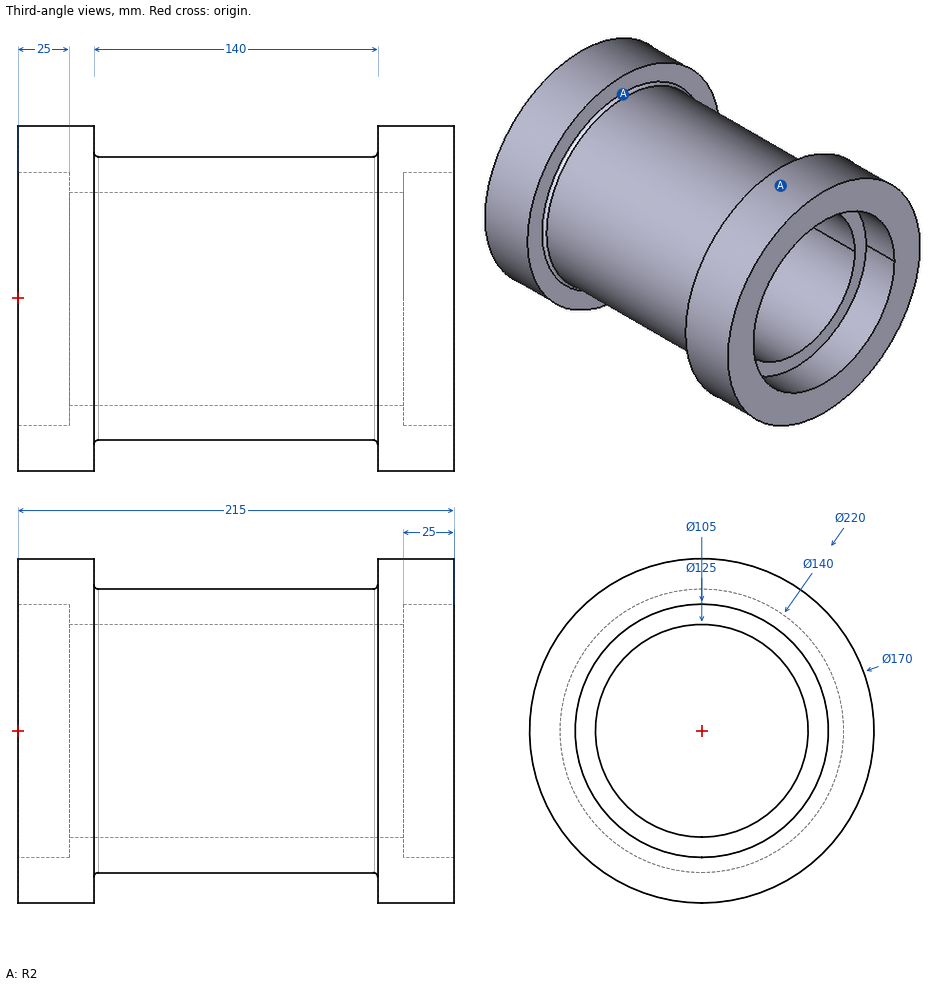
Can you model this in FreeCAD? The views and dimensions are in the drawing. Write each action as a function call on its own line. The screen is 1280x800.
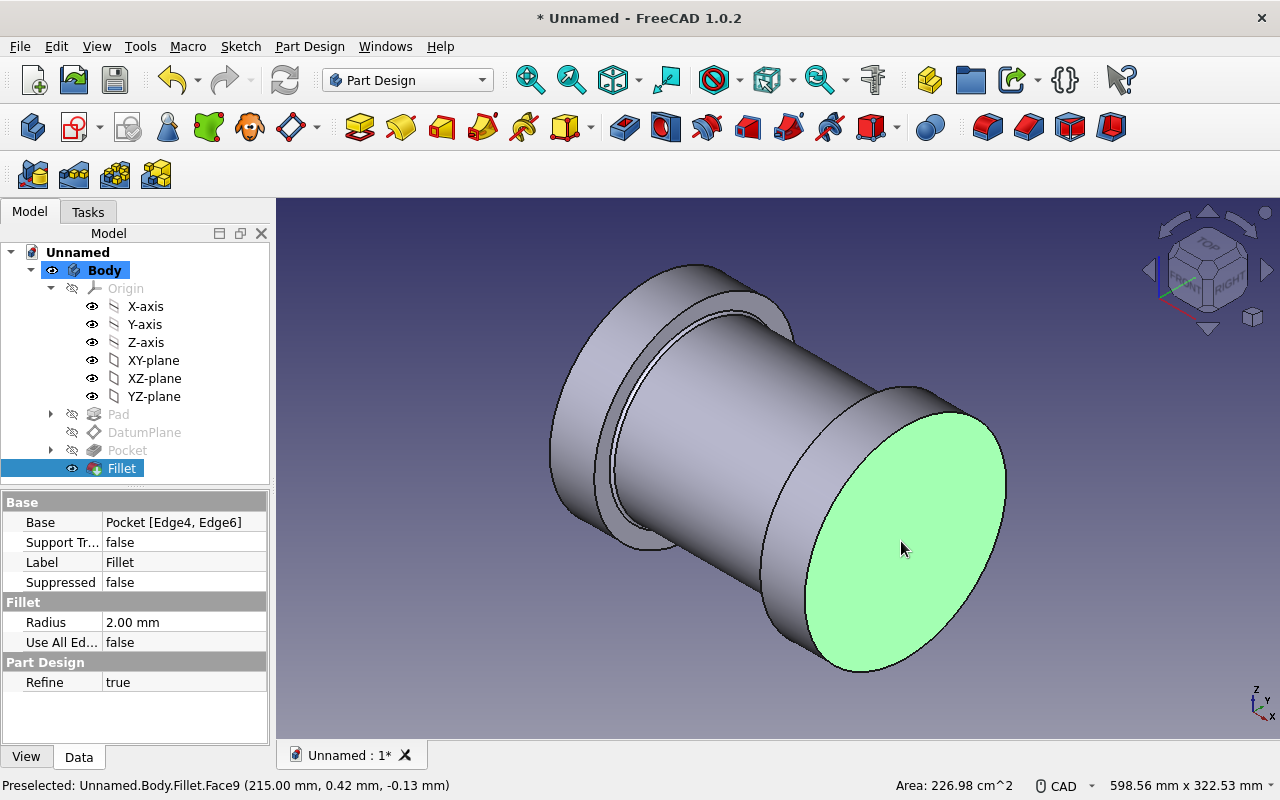
click(74, 128)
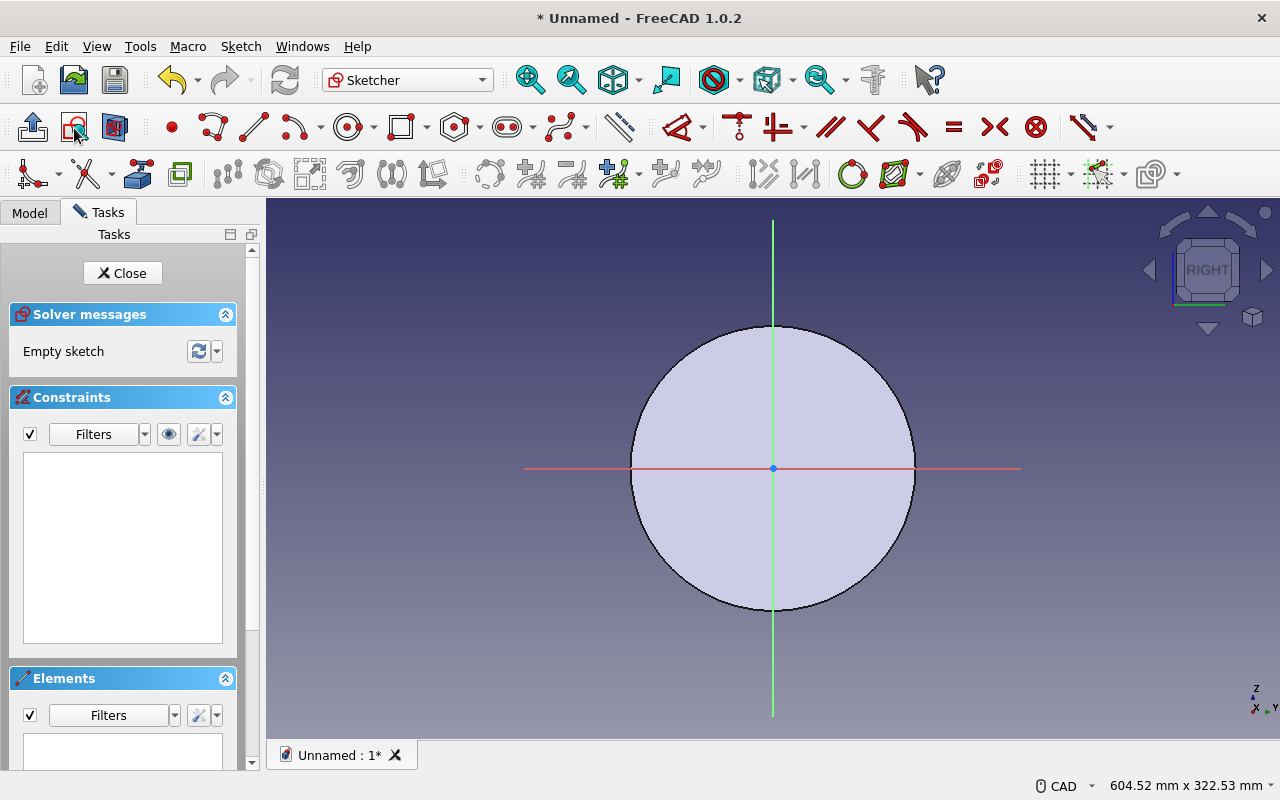
scroll(912, 468, up, 2)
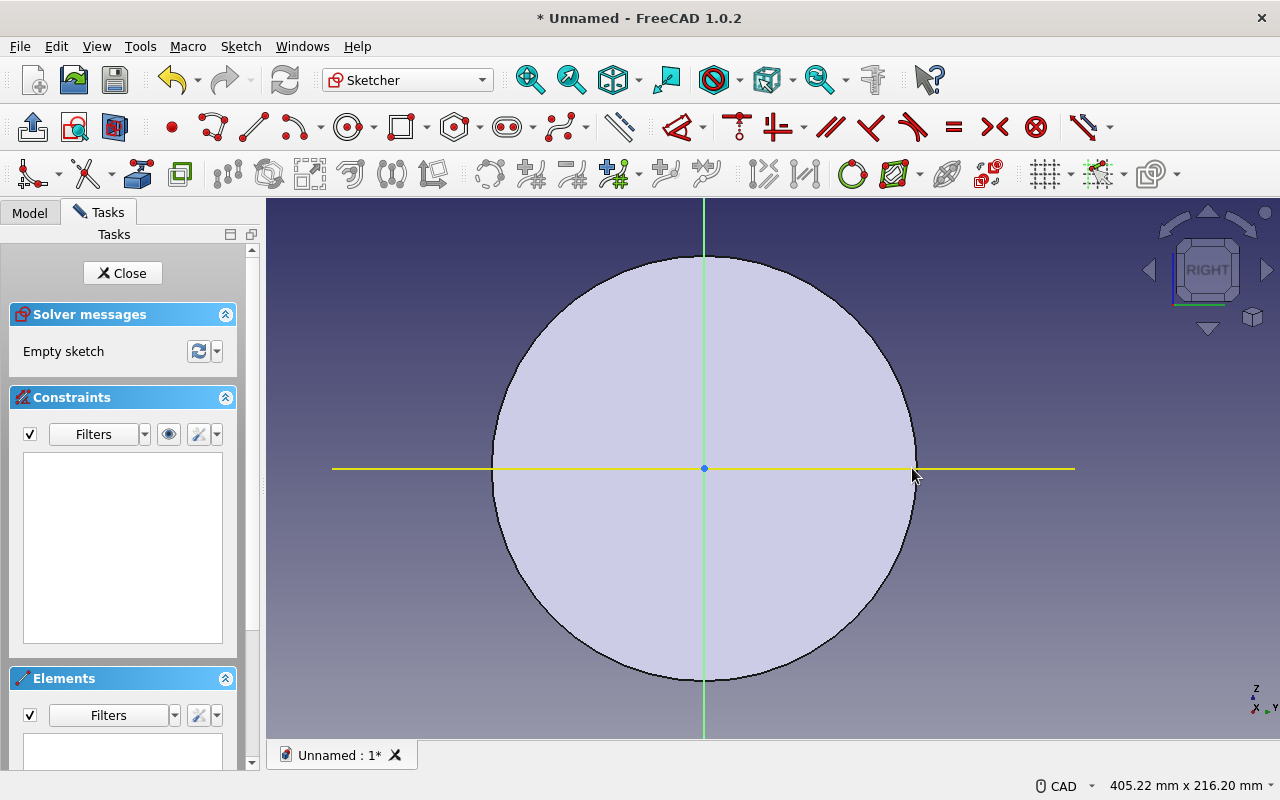
key(g)
key(c)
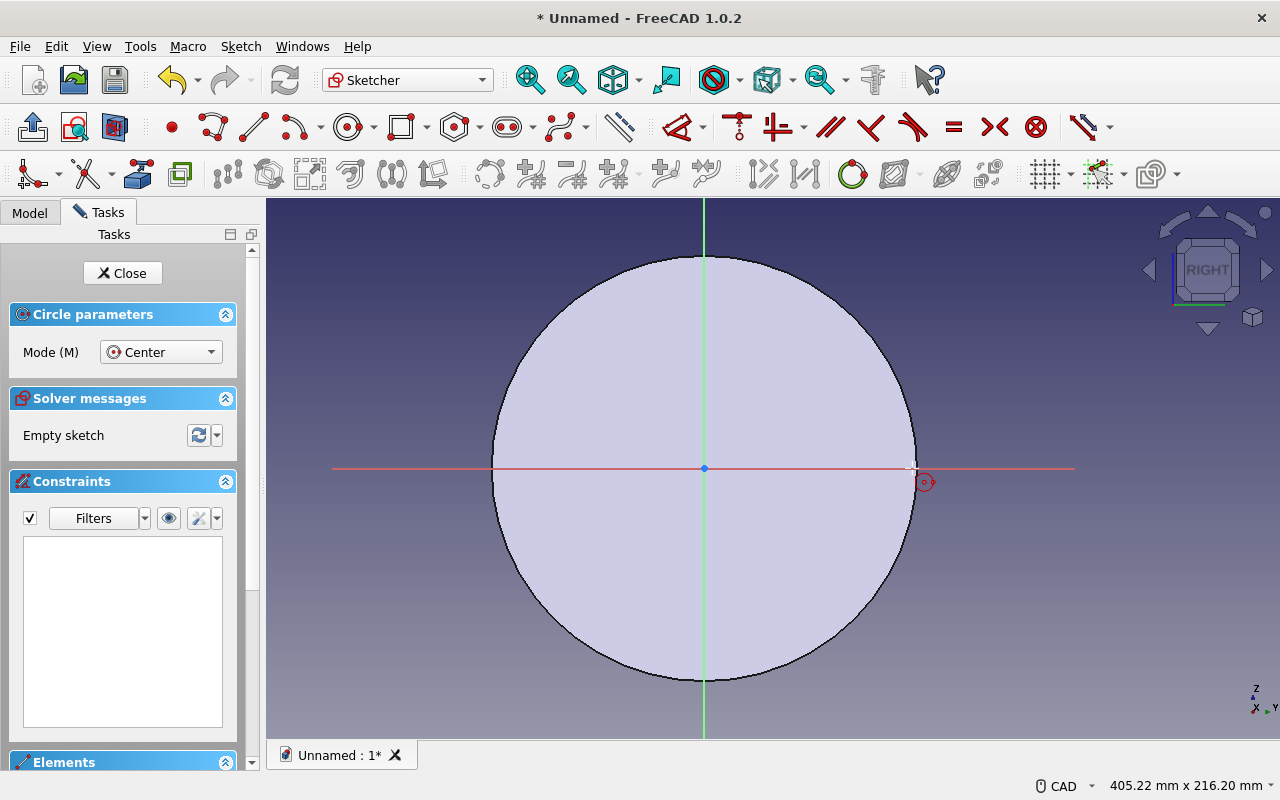
click(704, 468)
move(815, 358)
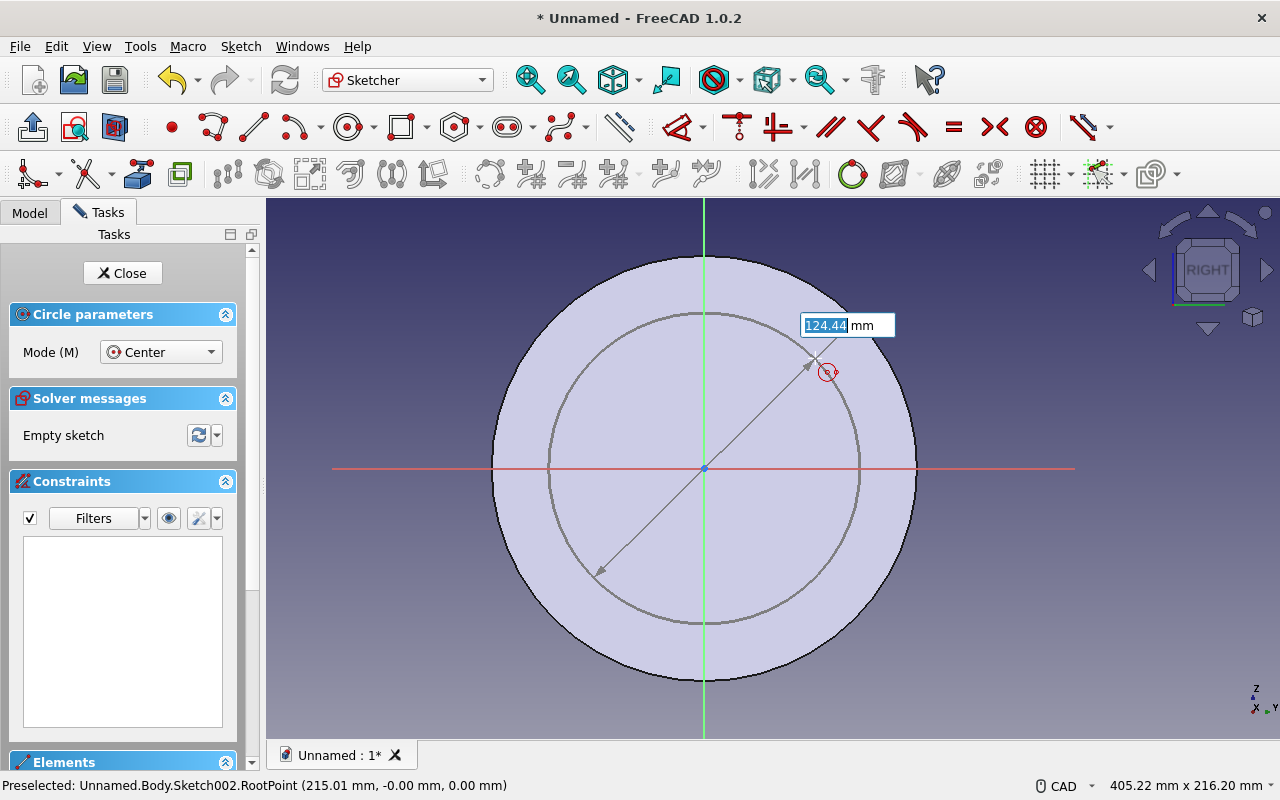
text(125)
key(Return)
key(Escape)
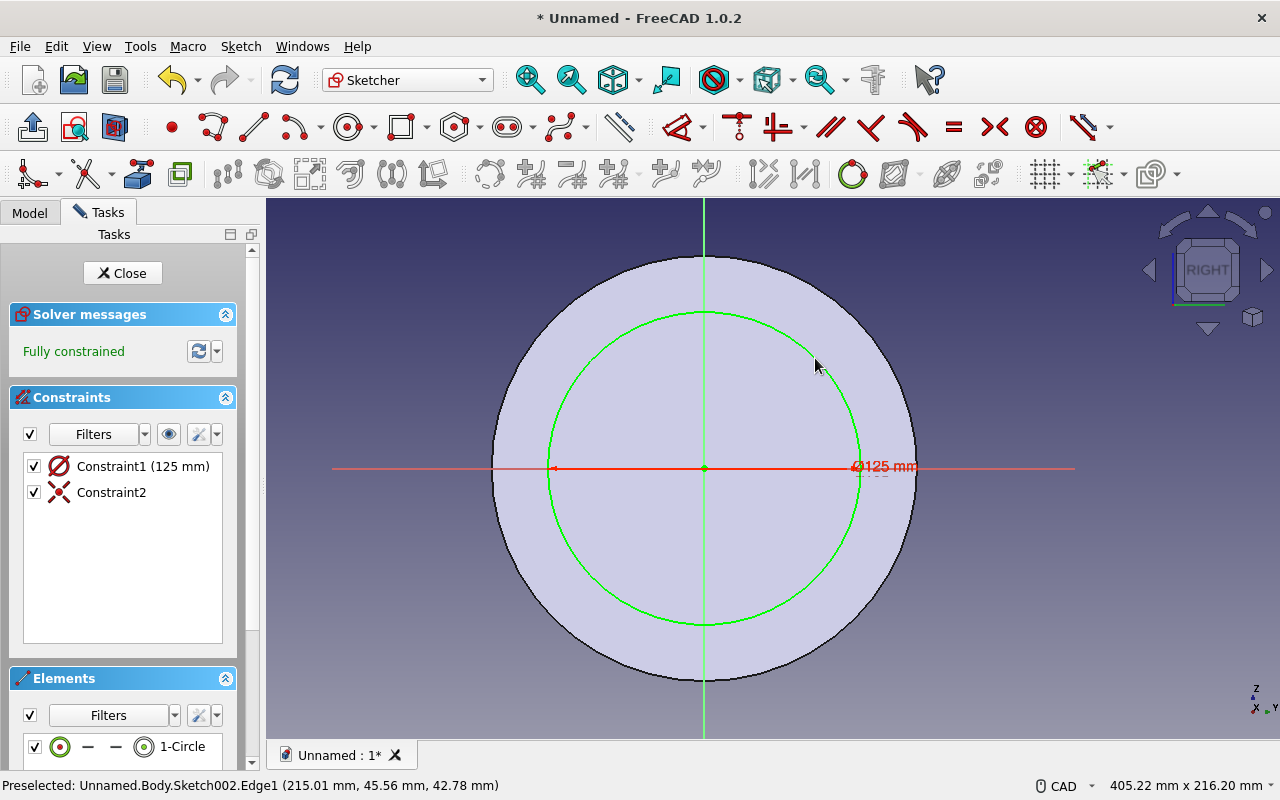
click(123, 273)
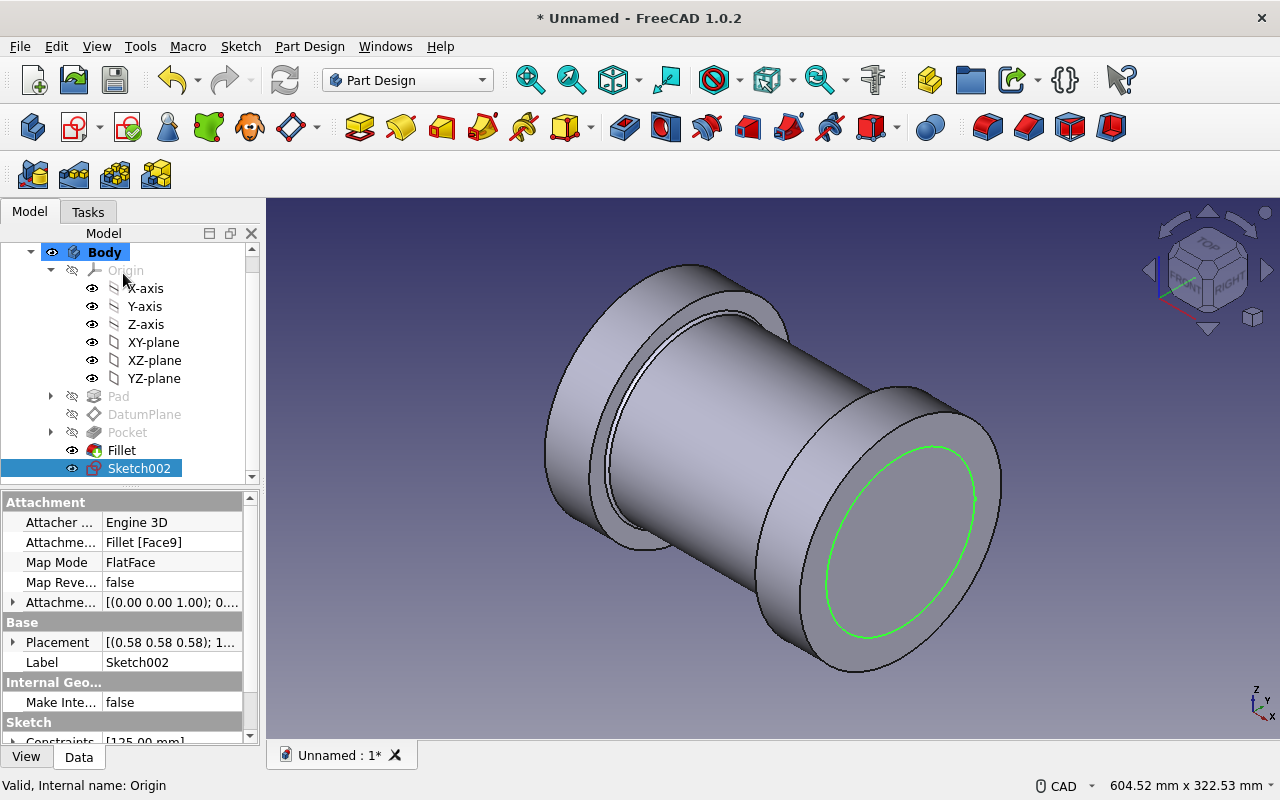
click(625, 128)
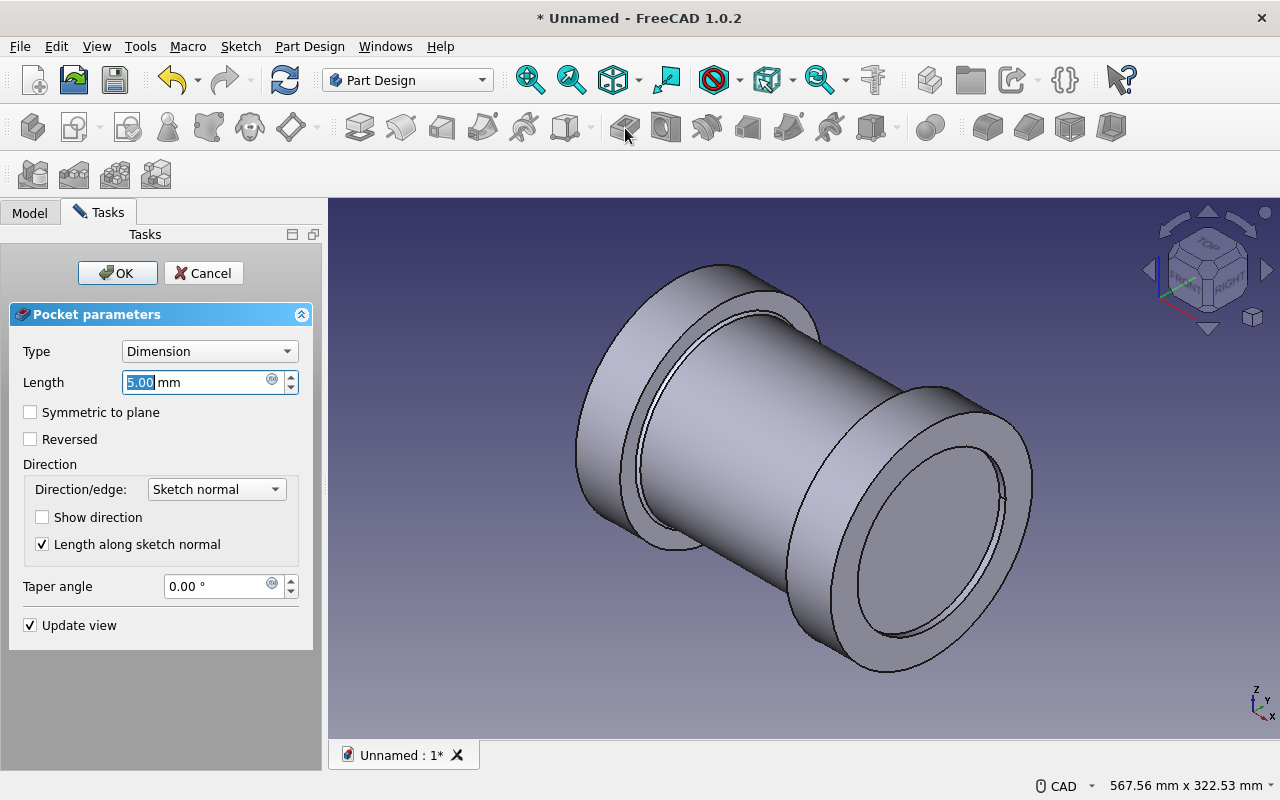
text(25)
key(Tab)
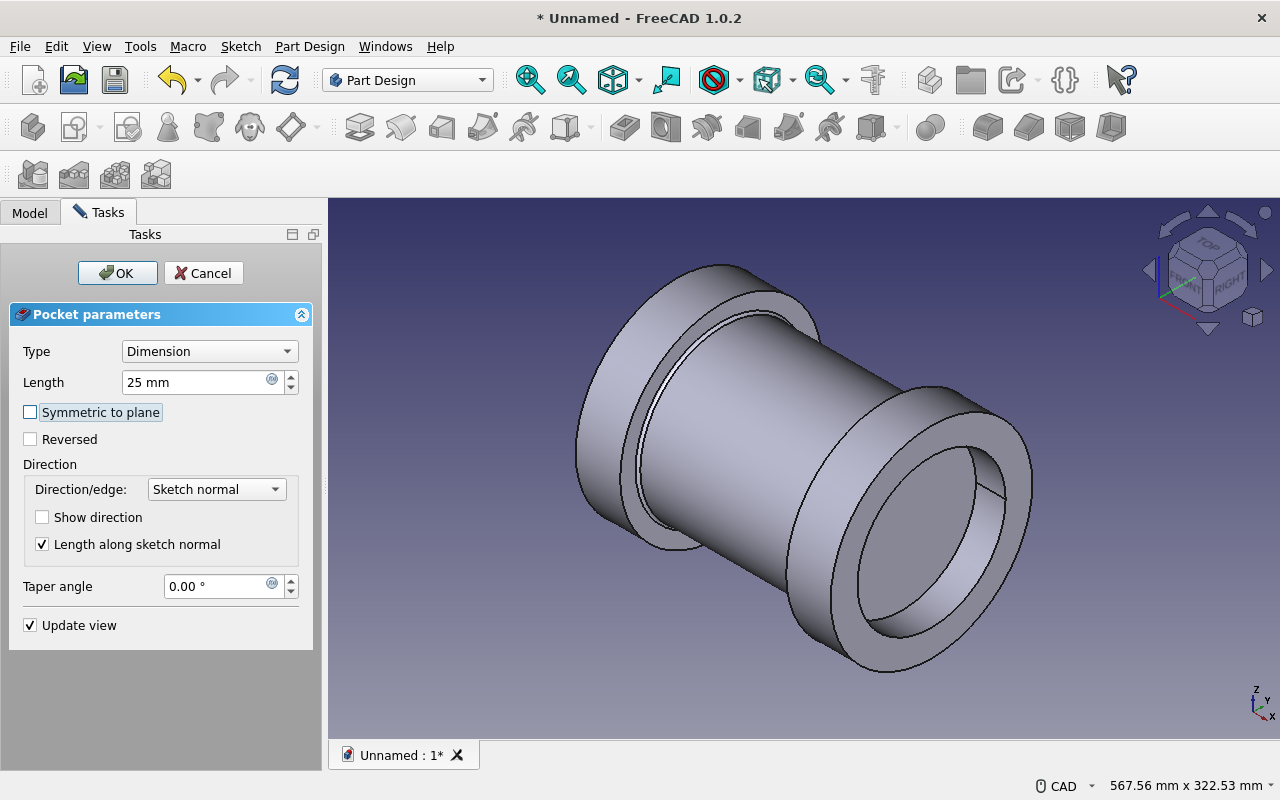
click(118, 273)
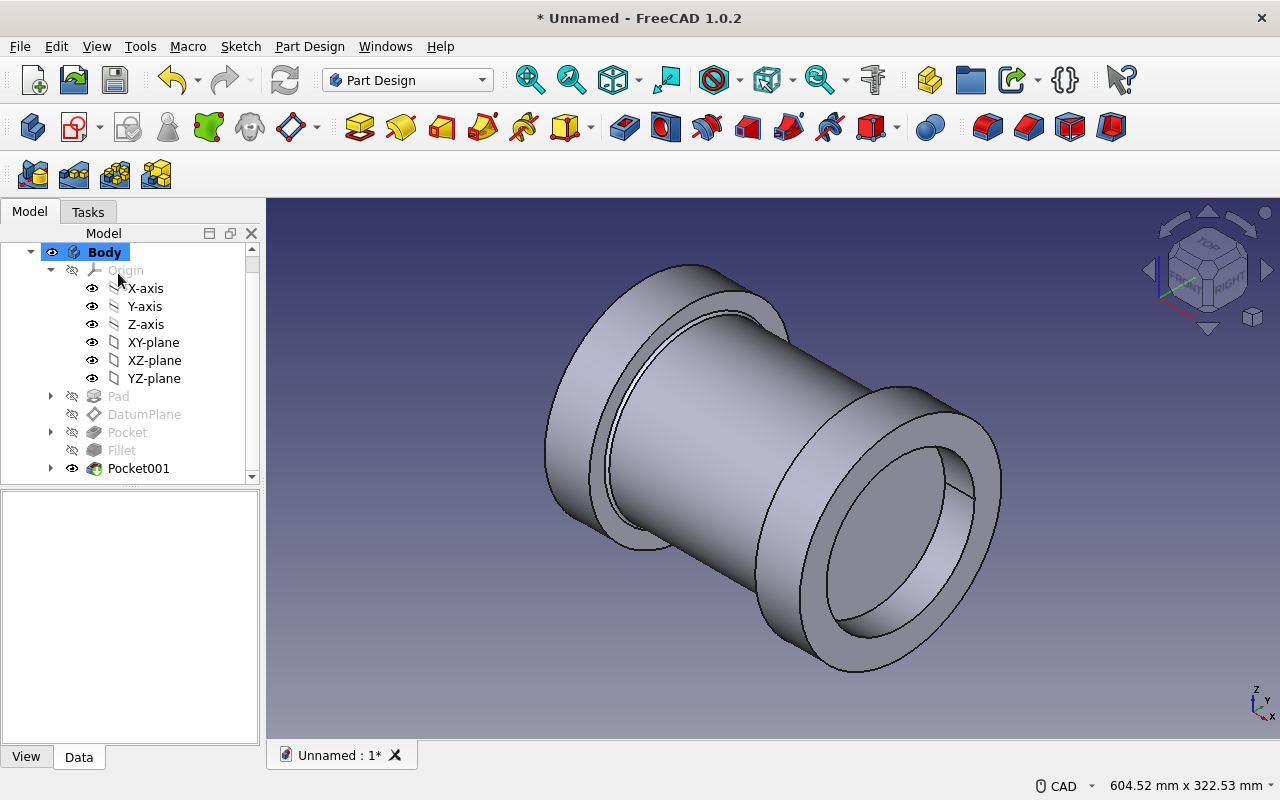
click(137, 378)